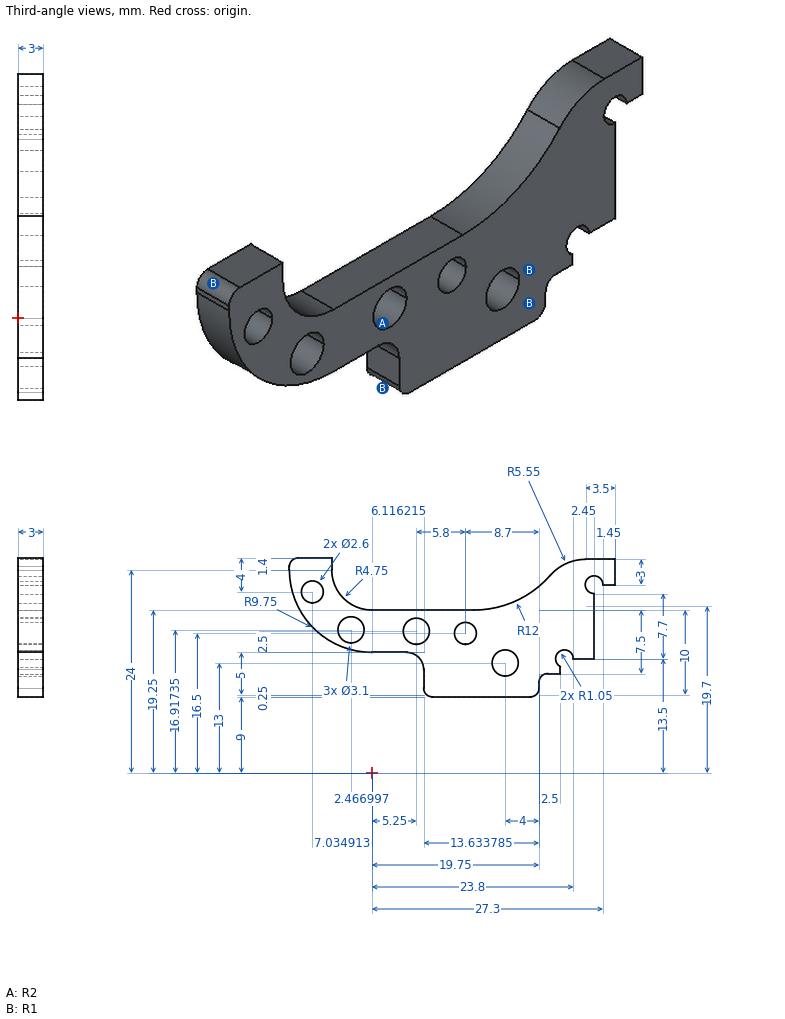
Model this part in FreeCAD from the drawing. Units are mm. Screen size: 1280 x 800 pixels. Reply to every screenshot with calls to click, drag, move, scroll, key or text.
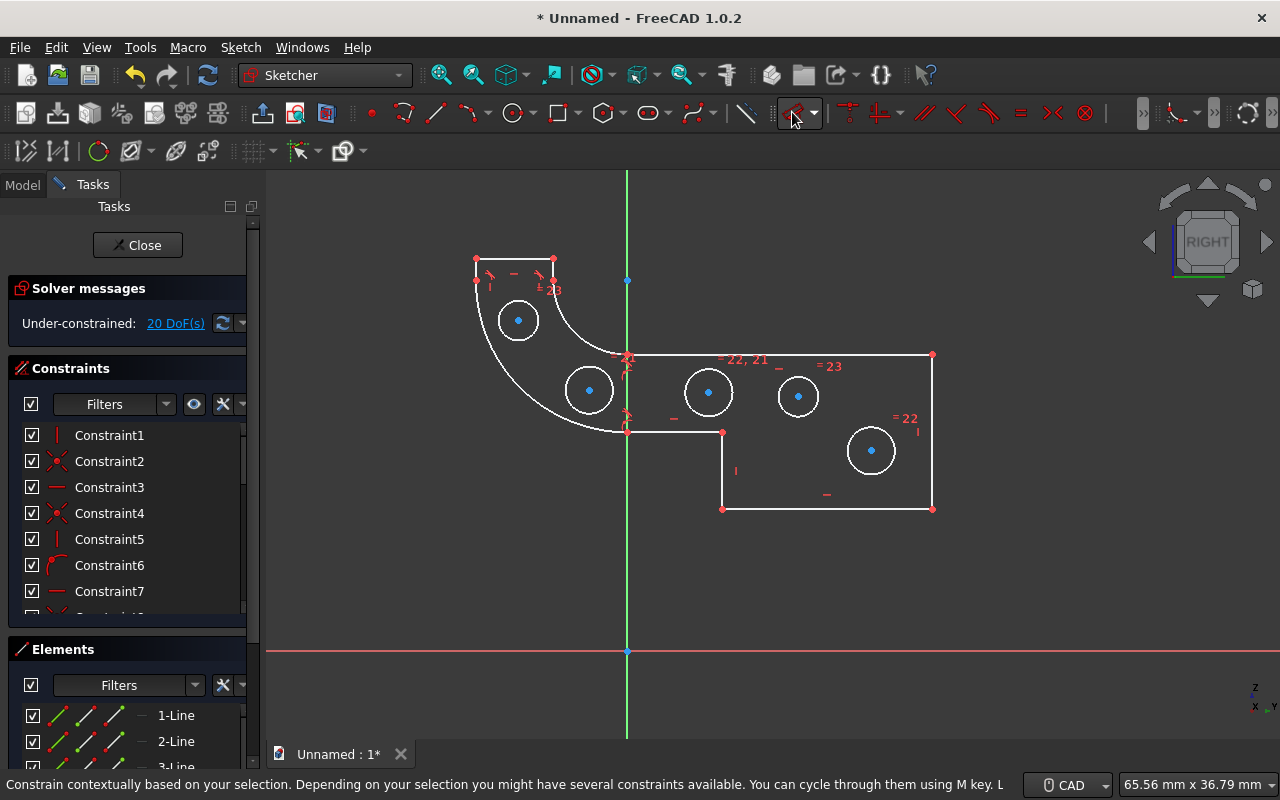
click(493, 350)
click(465, 365)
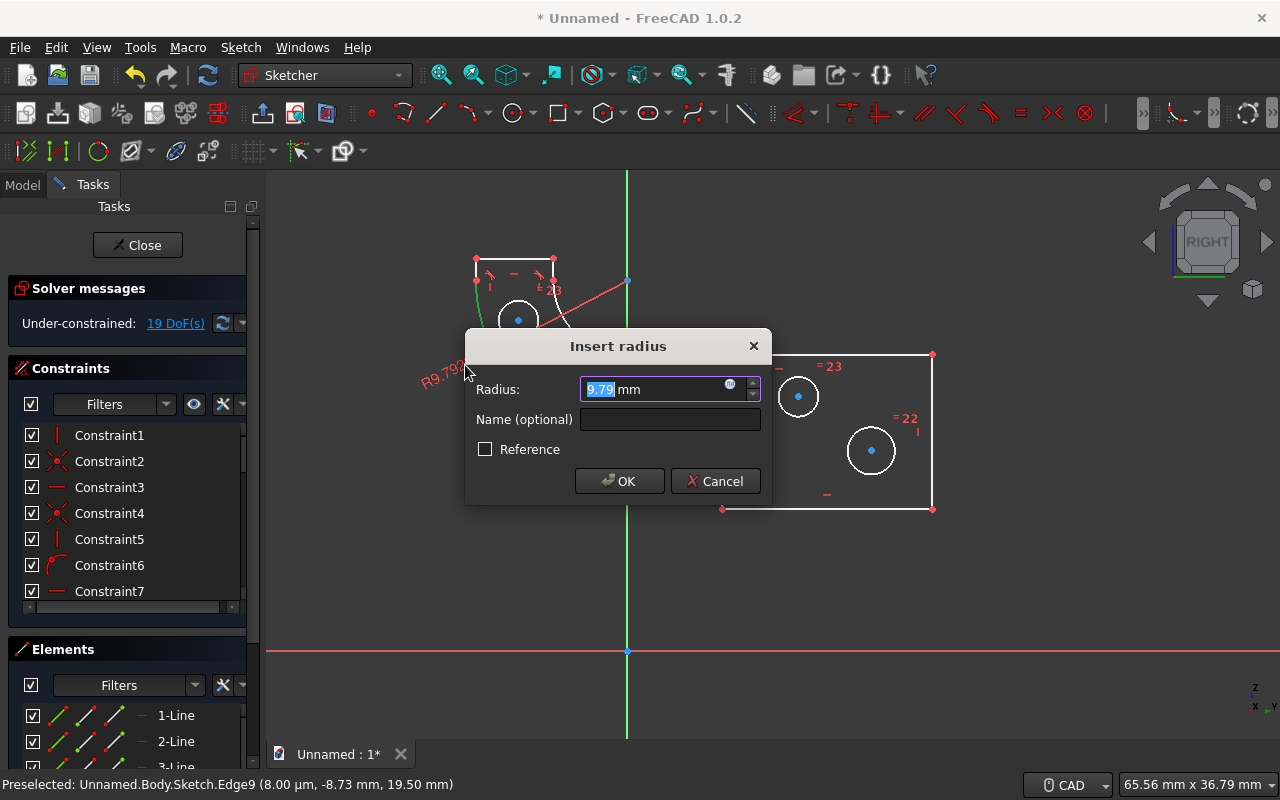
text(9.75)
key(Return)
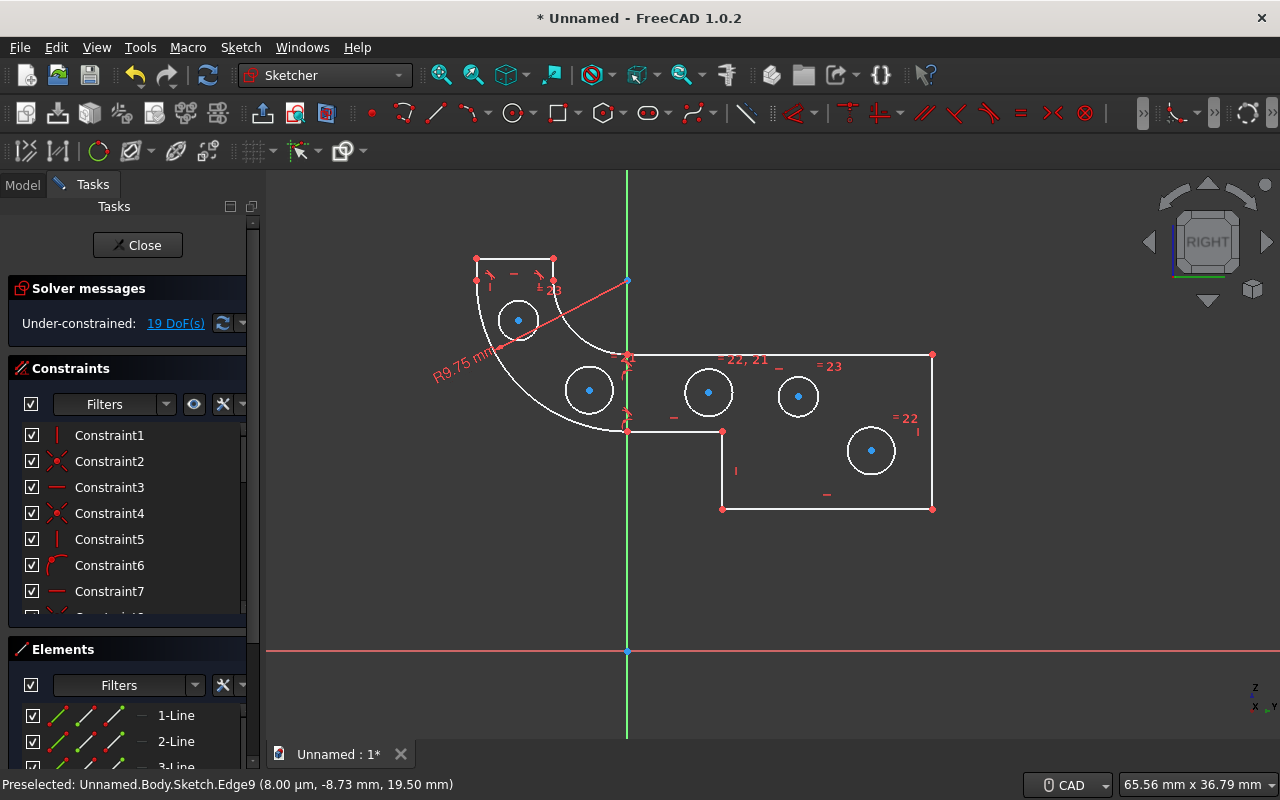
click(561, 314)
click(521, 277)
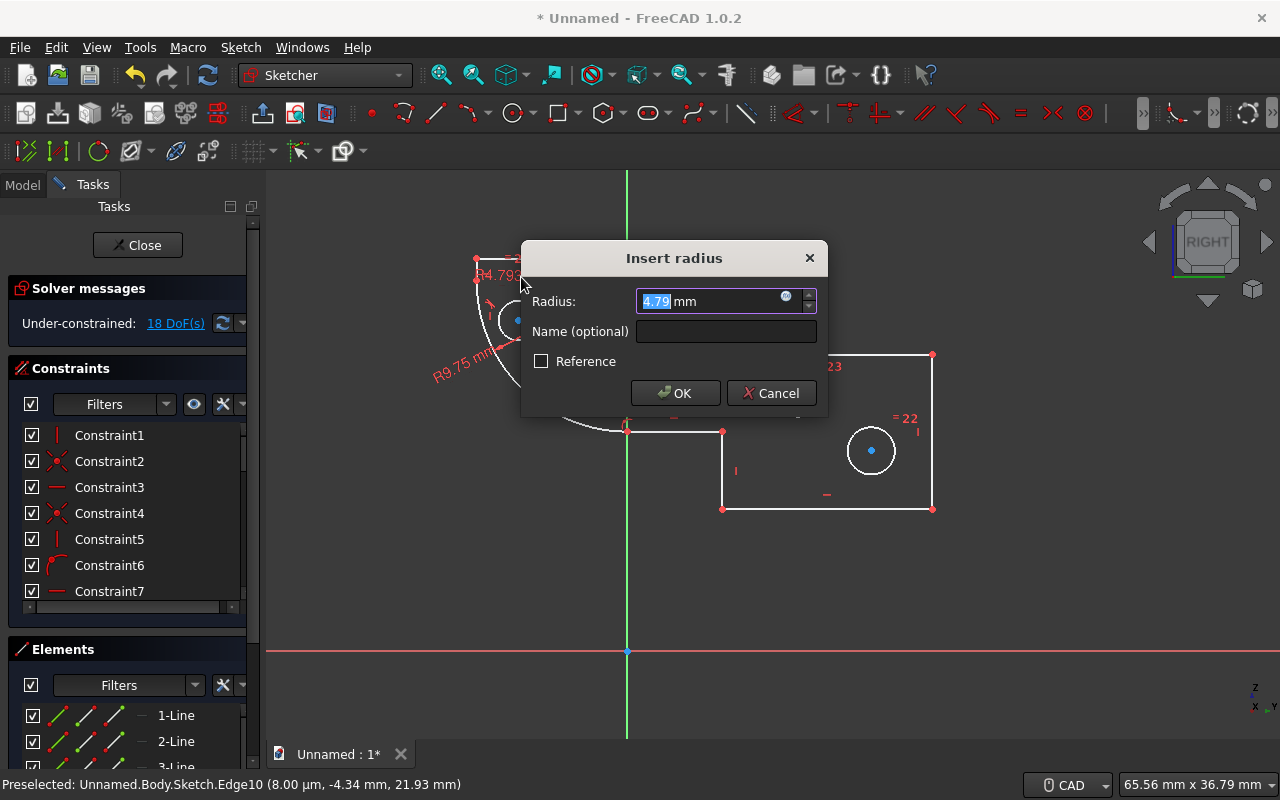
text(4.75)
key(Return)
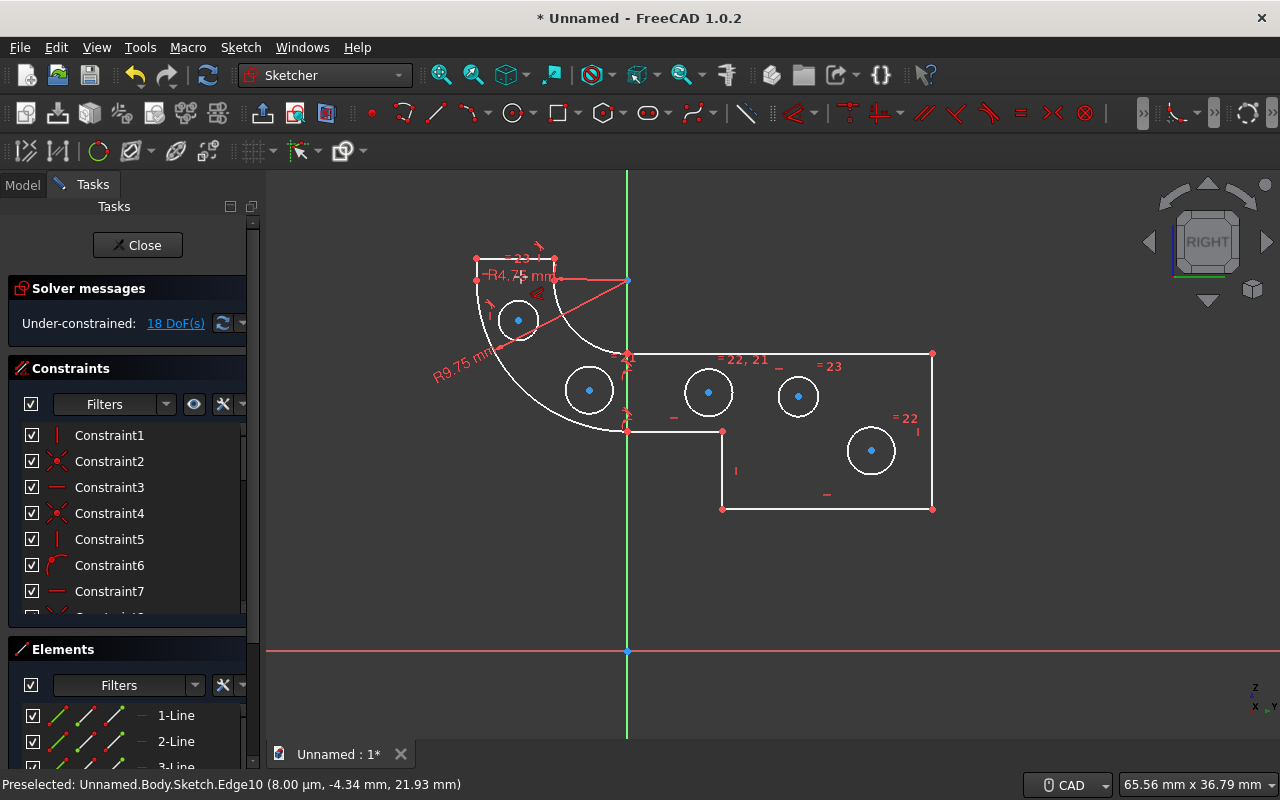
click(533, 307)
click(554, 358)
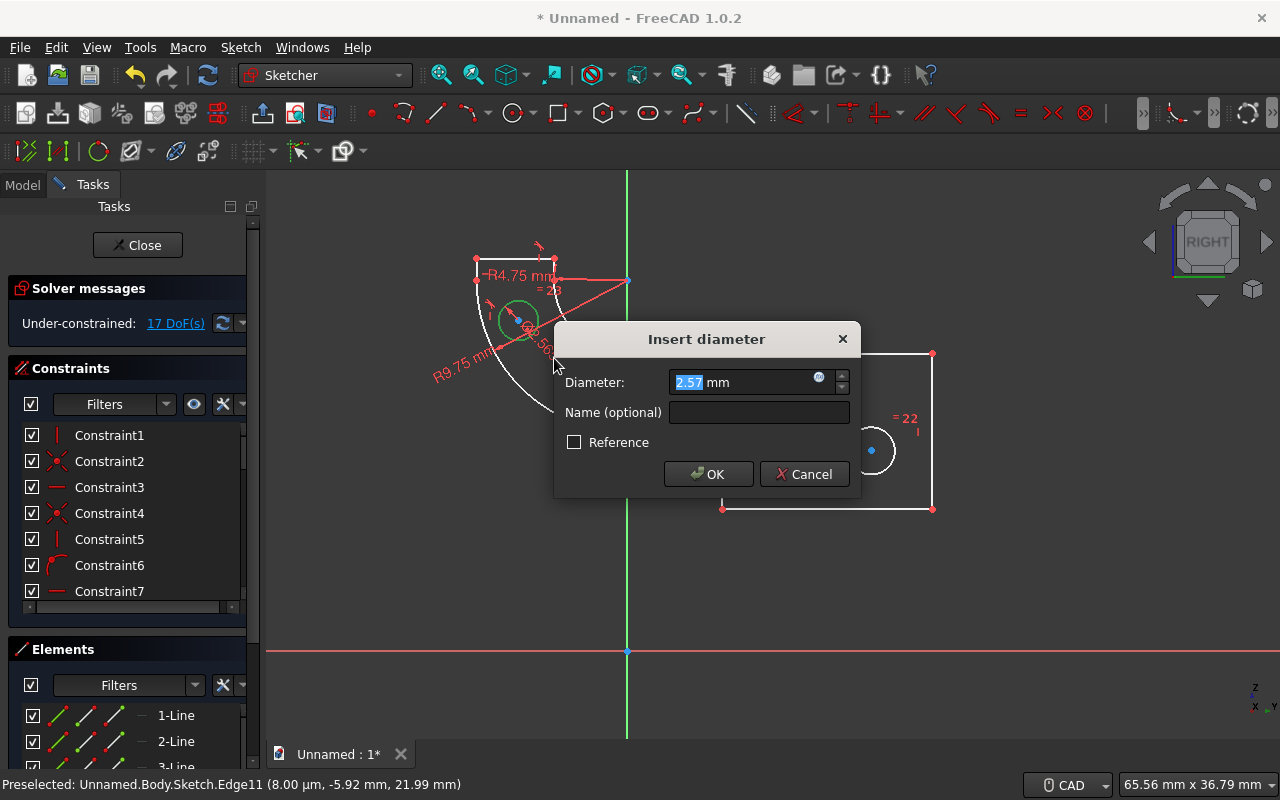
text(2.6)
key(Return)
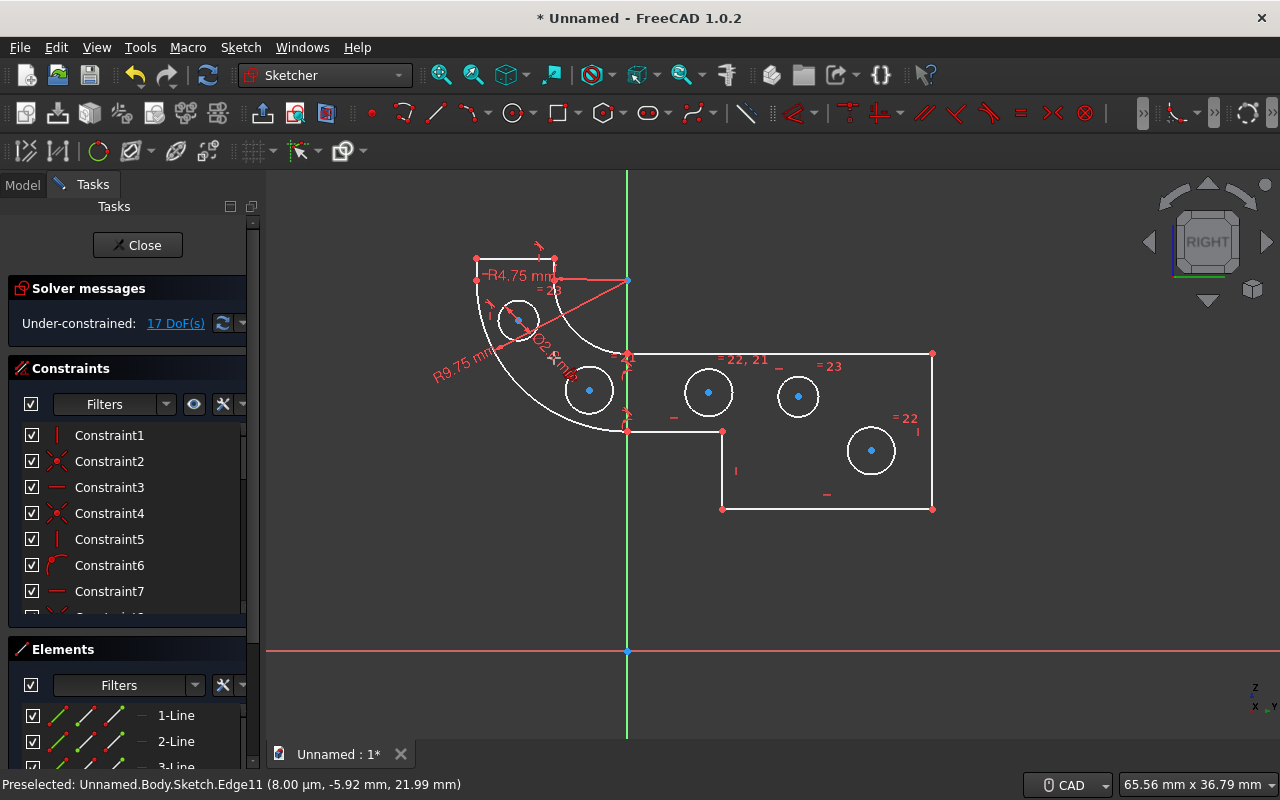
click(606, 373)
click(643, 374)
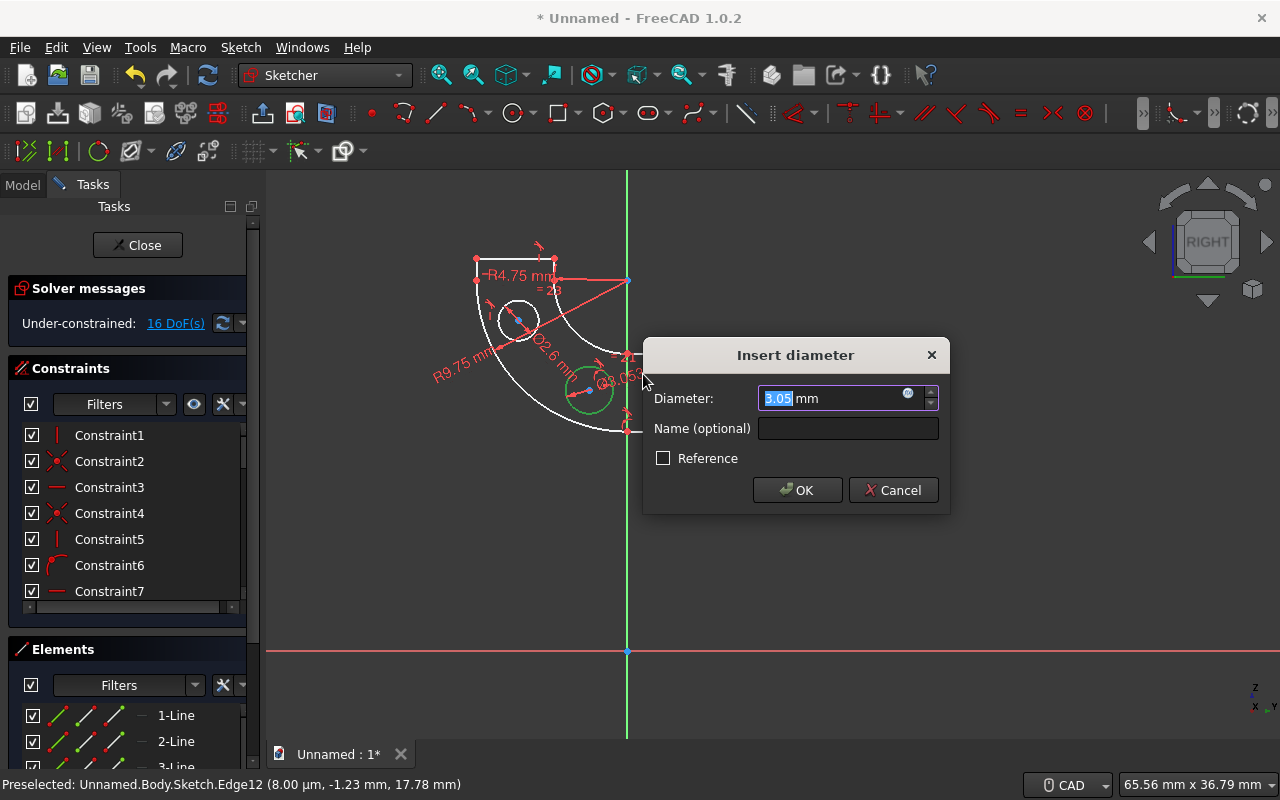
text(3.1)
key(Return)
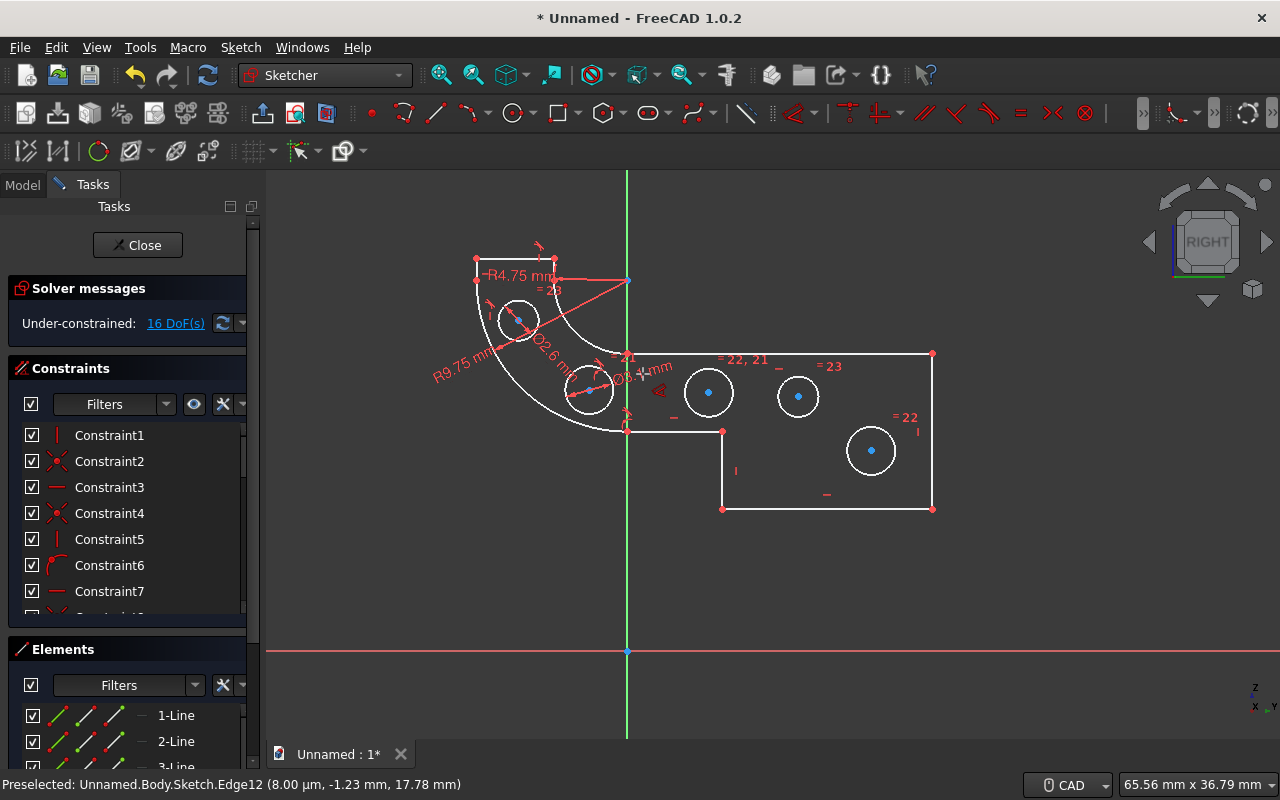
click(722, 455)
click(756, 470)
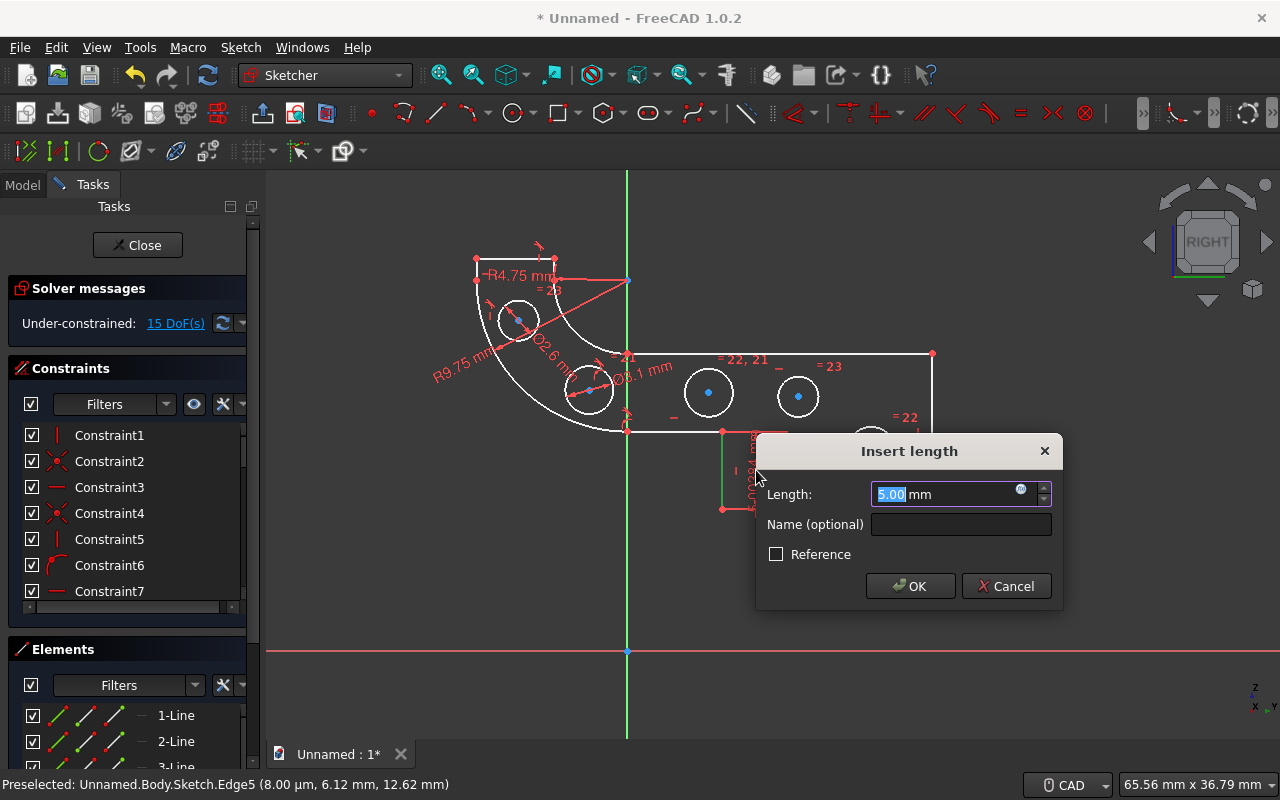
text(5)
key(Return)